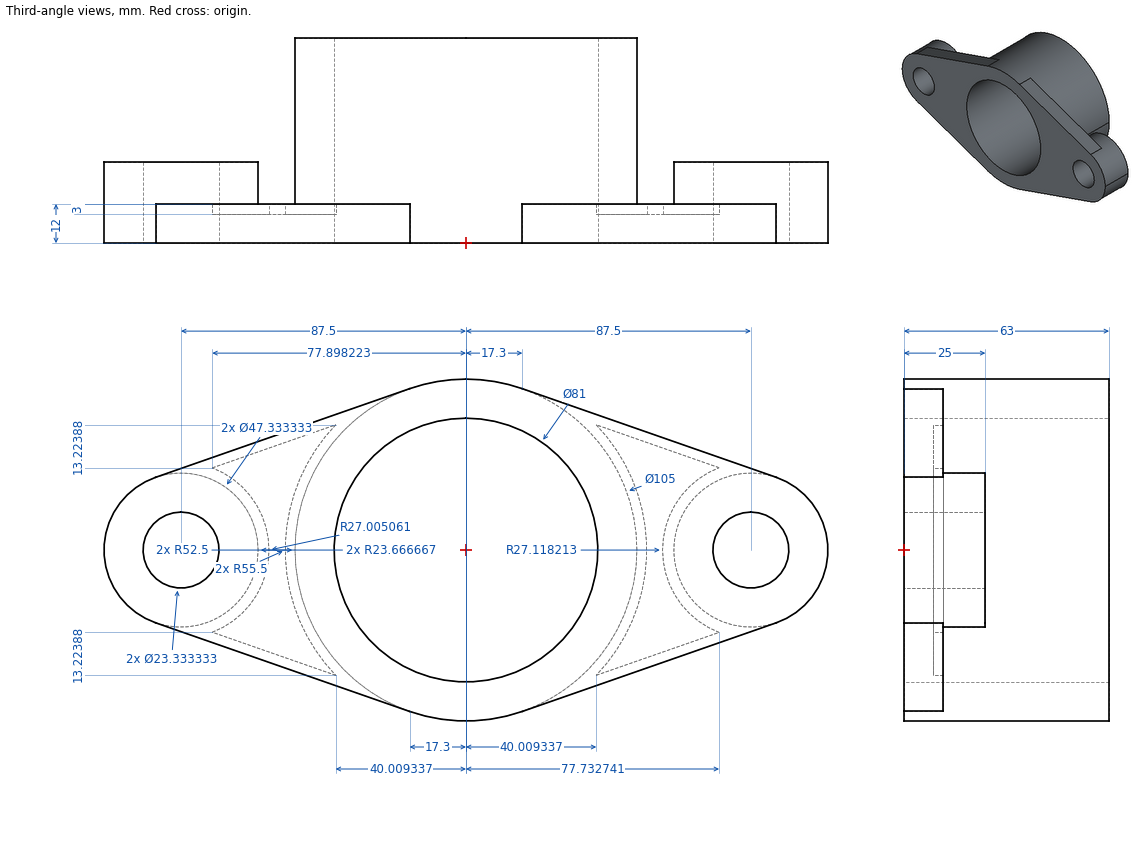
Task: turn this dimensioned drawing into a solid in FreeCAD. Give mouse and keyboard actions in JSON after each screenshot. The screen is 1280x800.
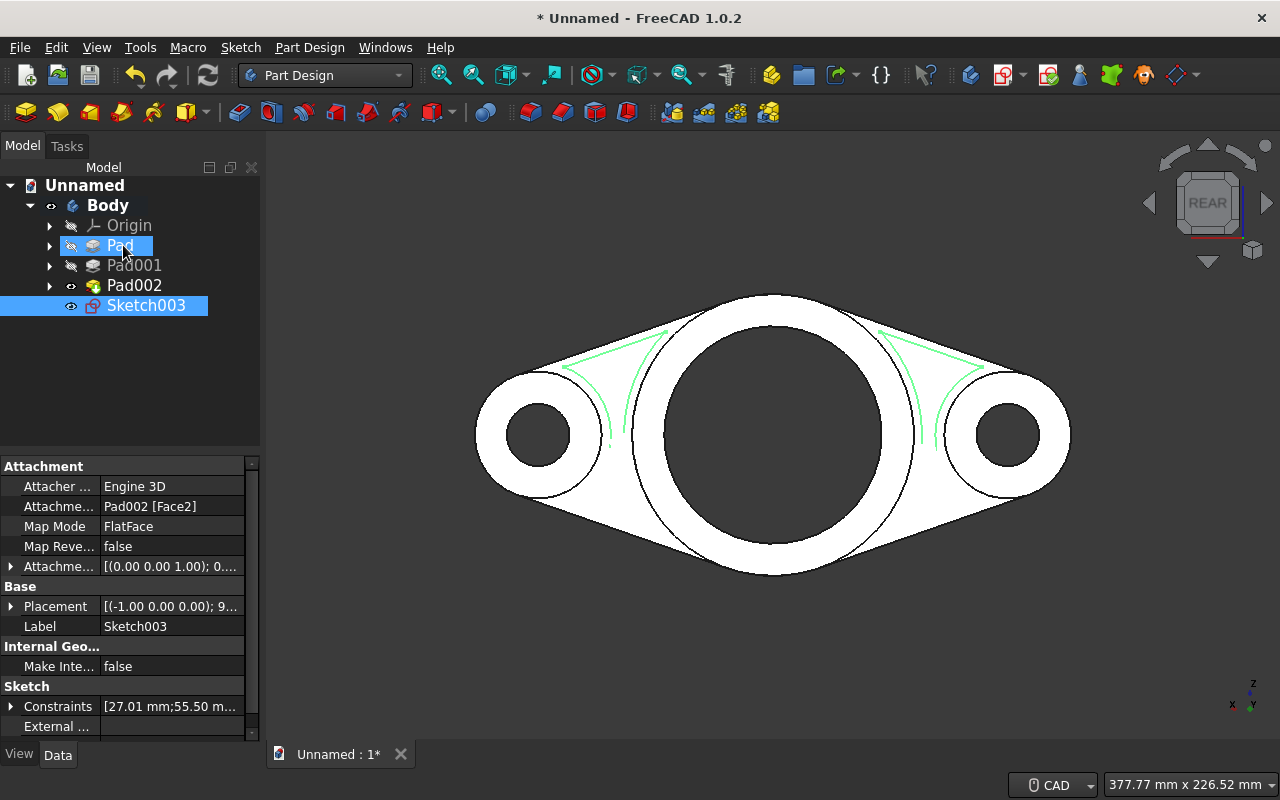
{"action": "left_click", "coordinate": [240, 112]}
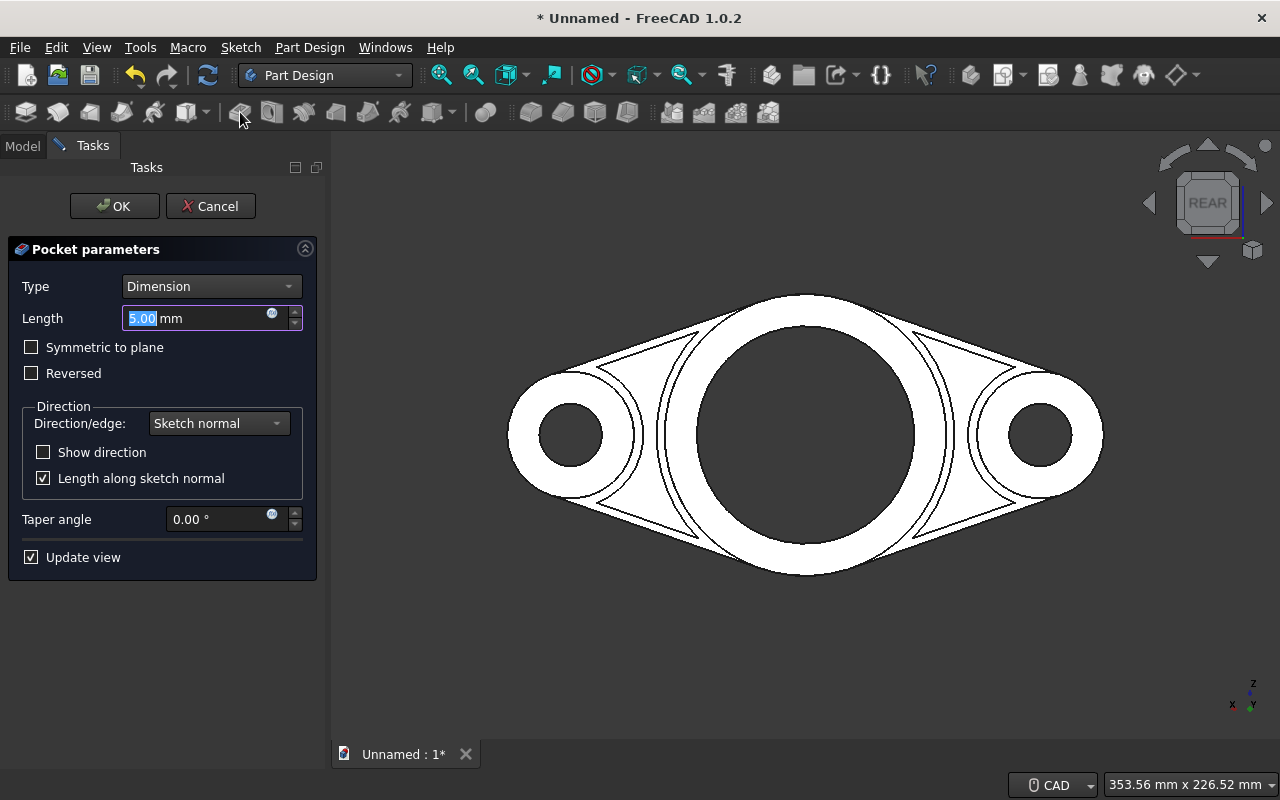
{"action": "type", "text": "3"}
{"action": "key", "text": "Tab"}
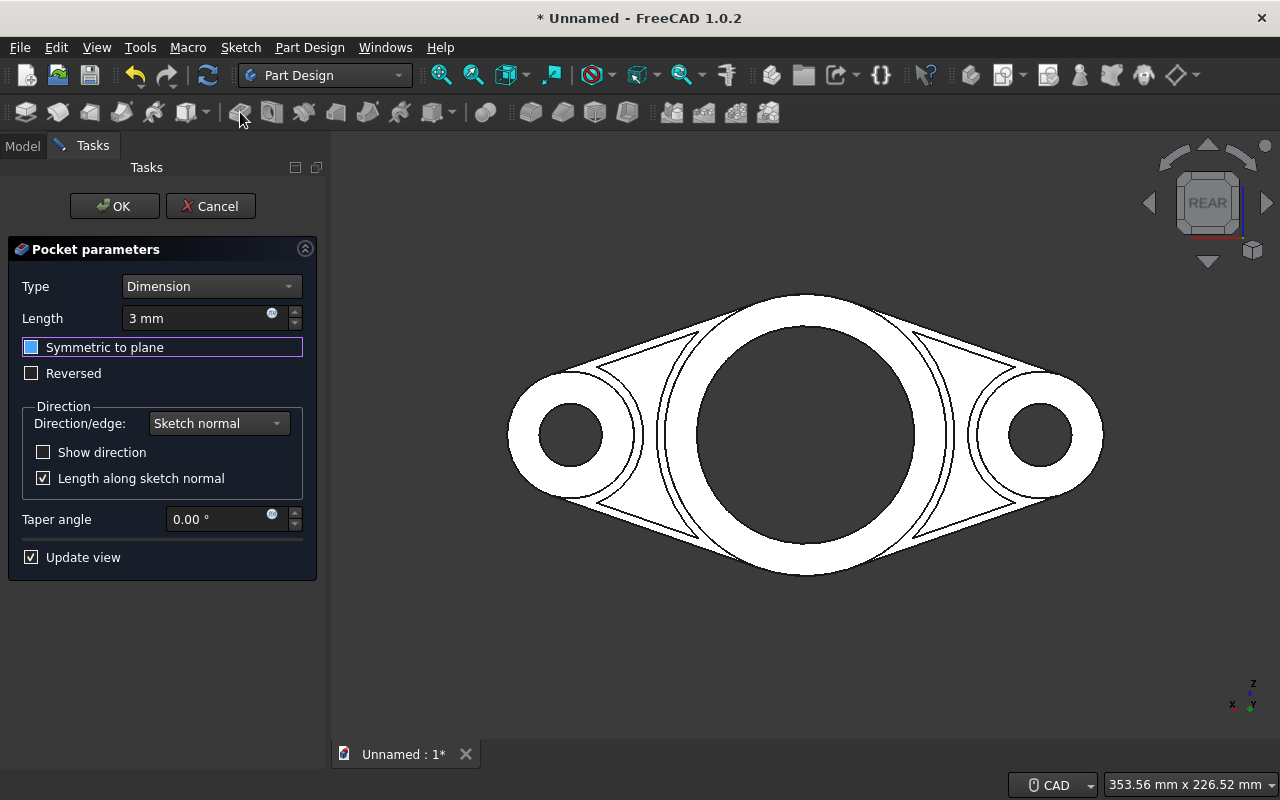
{"action": "left_click", "coordinate": [115, 206]}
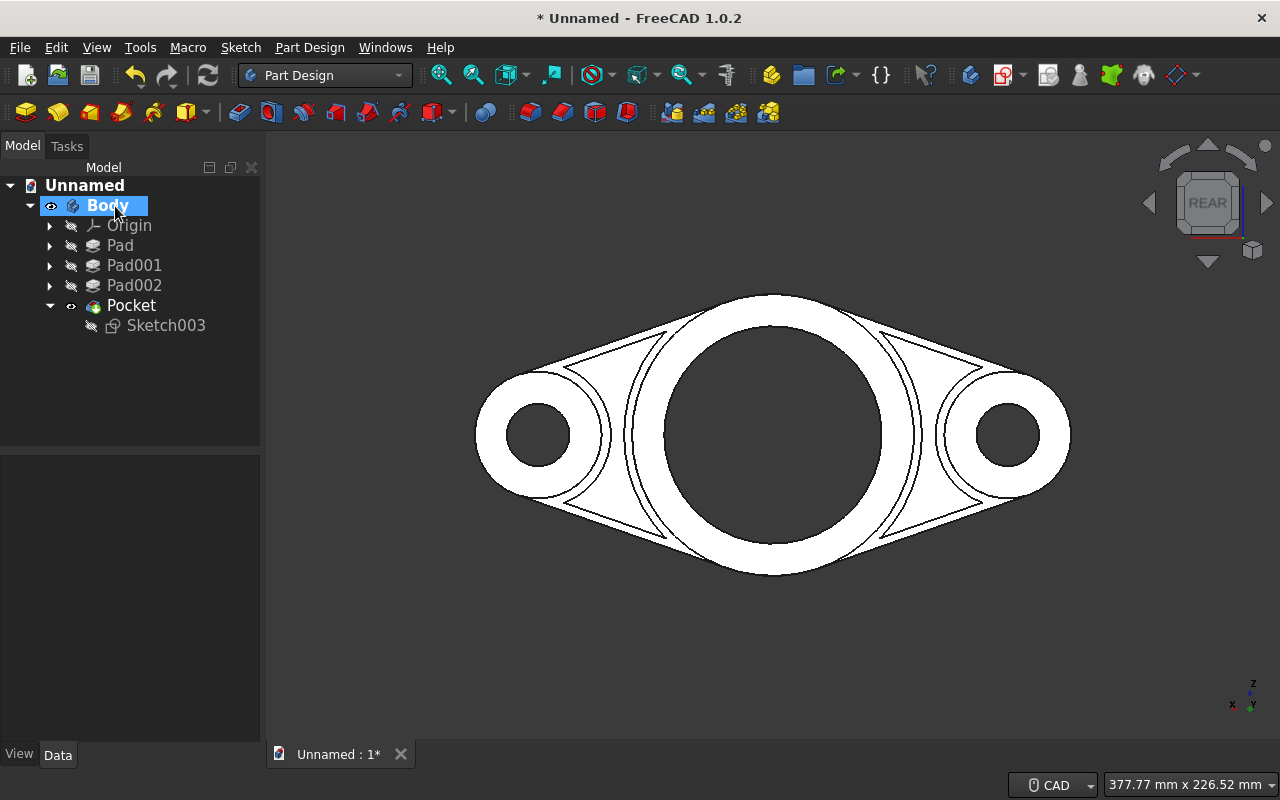
{"action": "key", "text": "0"}